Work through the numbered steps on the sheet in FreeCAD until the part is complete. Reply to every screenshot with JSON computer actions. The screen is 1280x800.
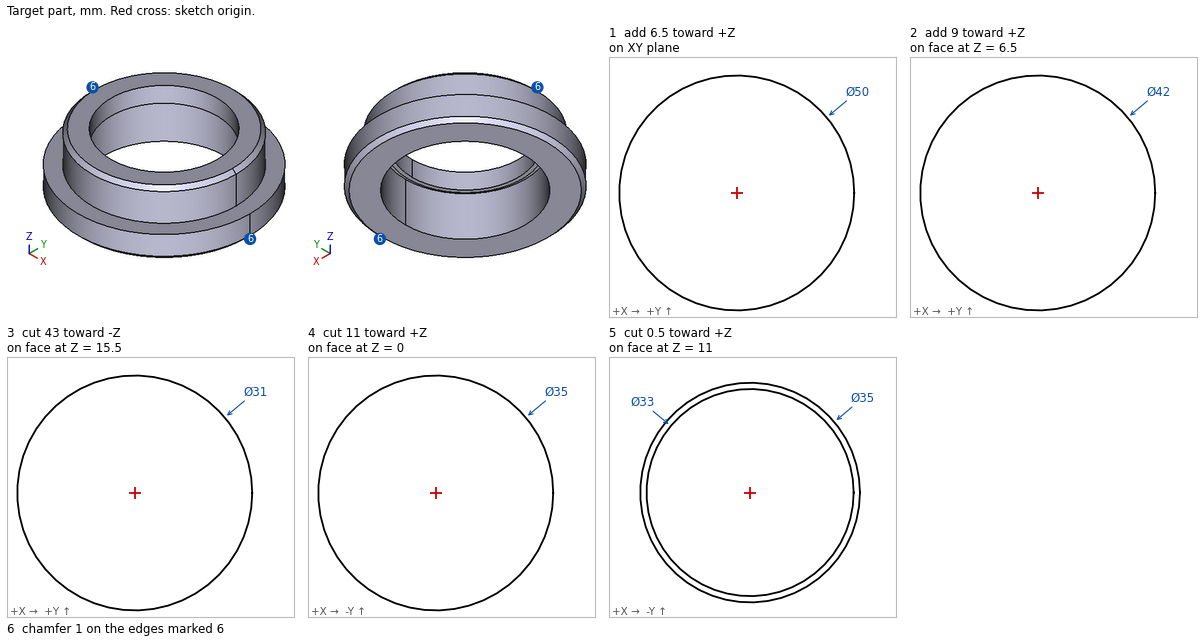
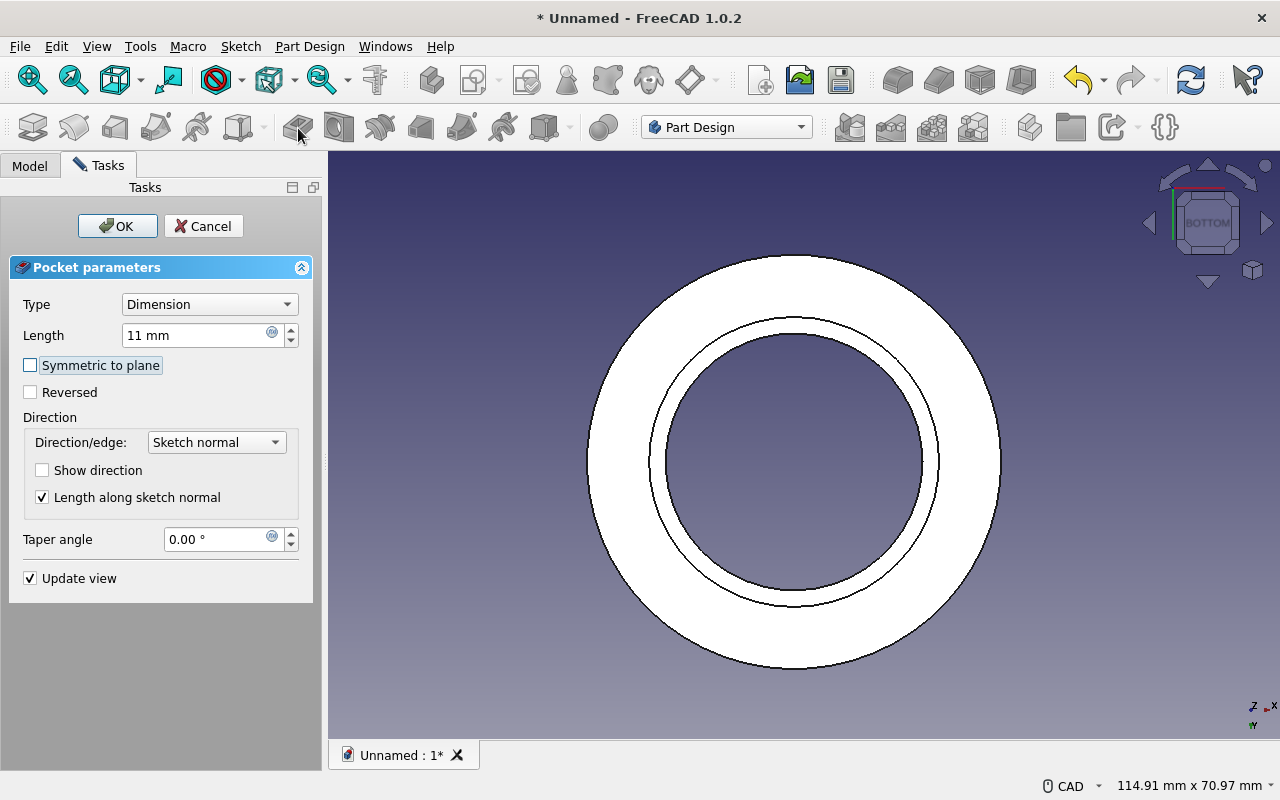
{"action": "left_click", "coordinate": [118, 226]}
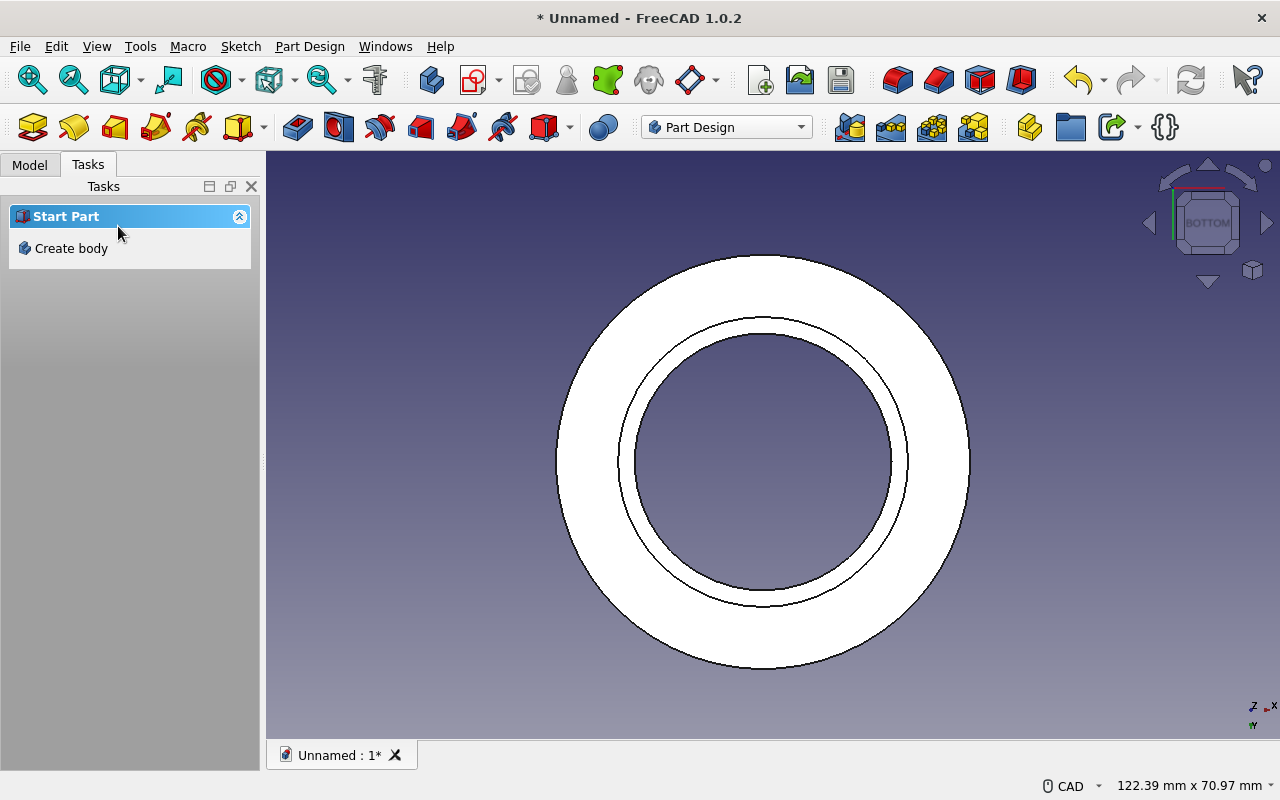
{"action": "scroll", "coordinate": [722, 337], "scroll_direction": "up", "scroll_amount": 8}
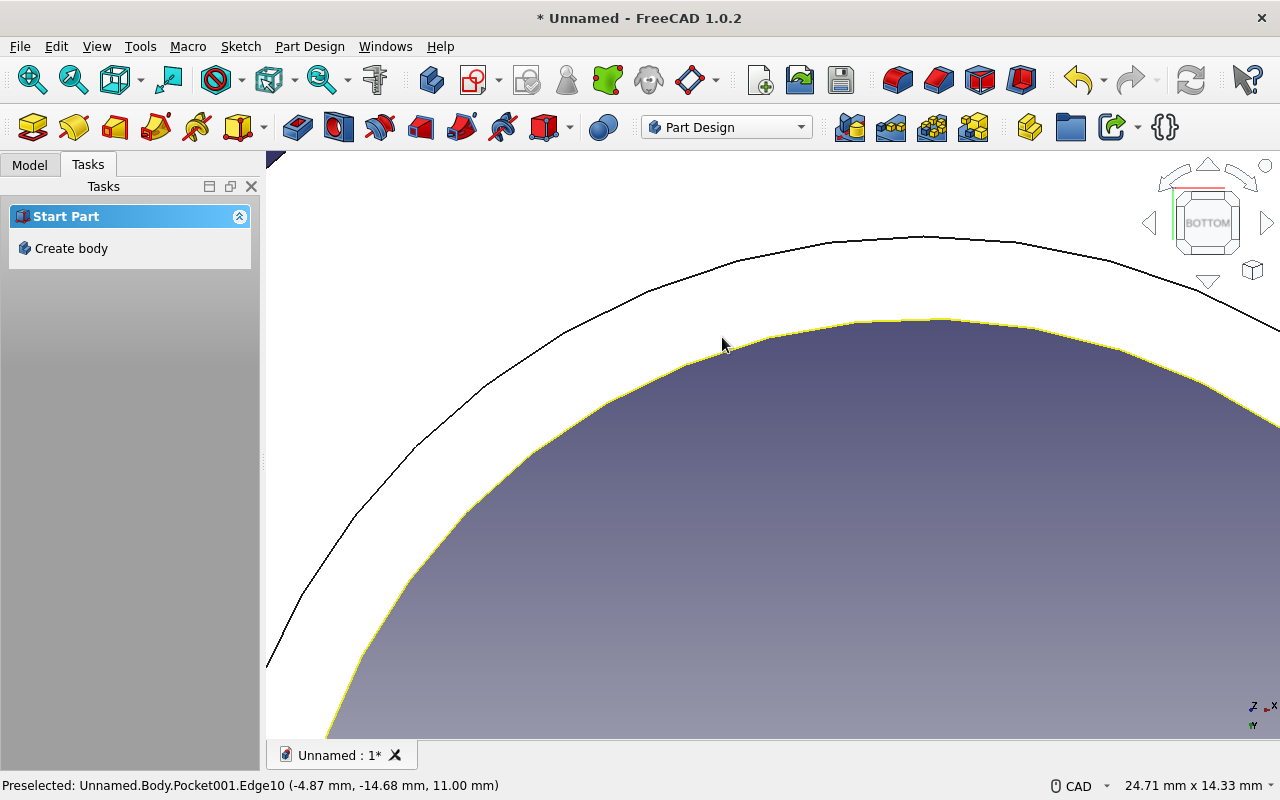
{"action": "left_click", "coordinate": [718, 338]}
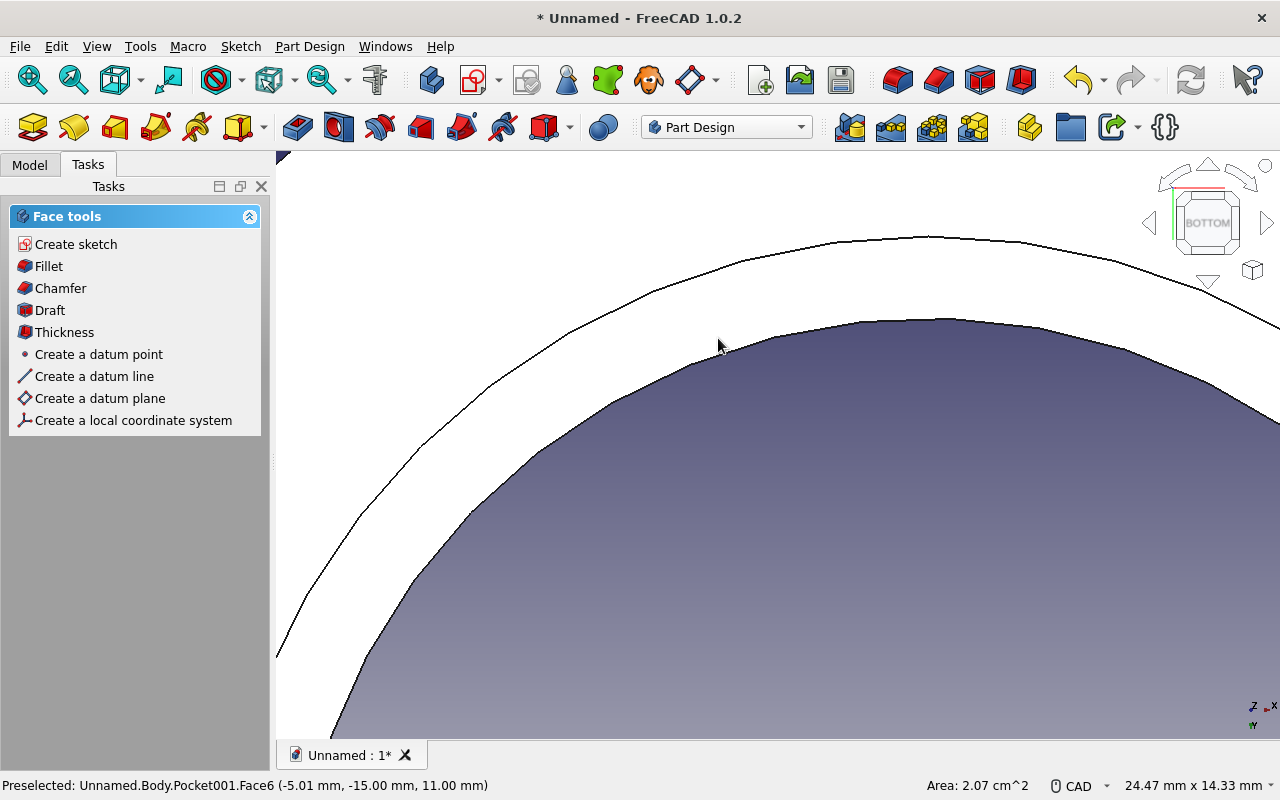
{"action": "left_click", "coordinate": [472, 80]}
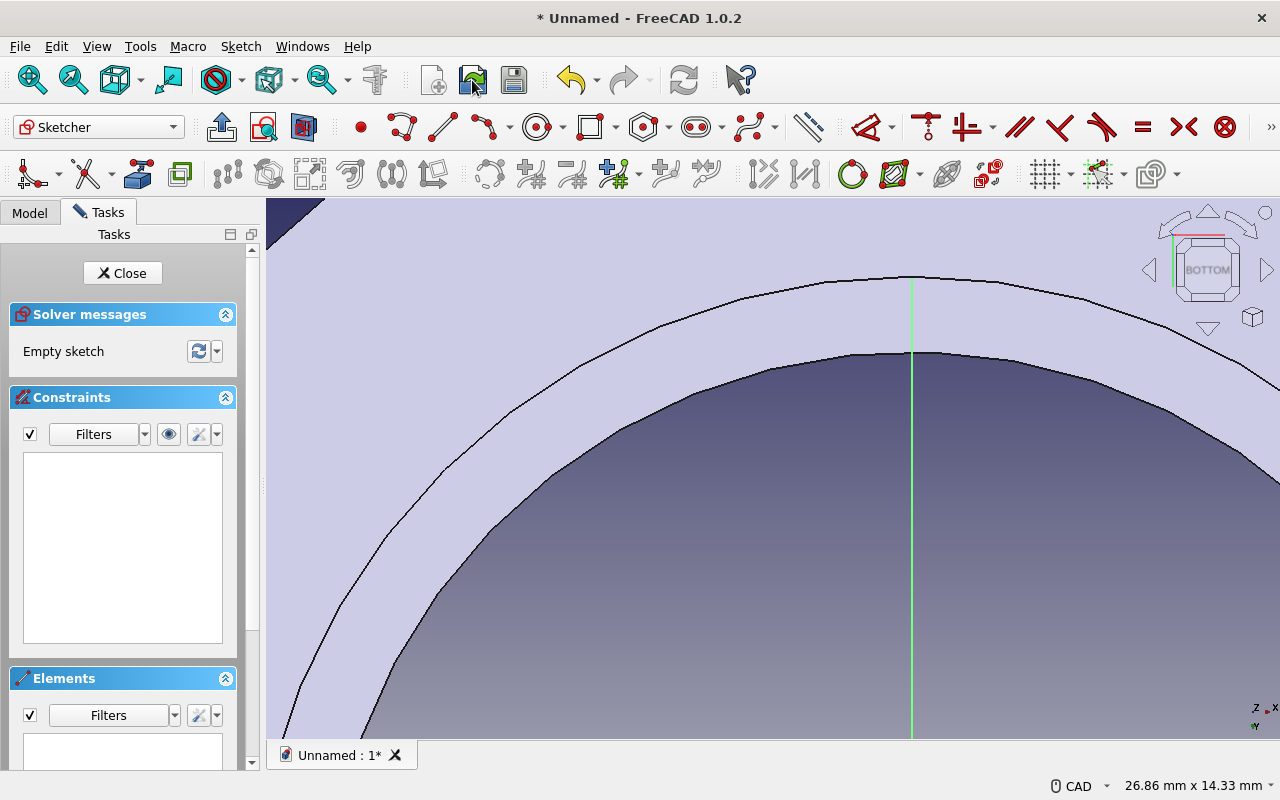
{"action": "left_click", "coordinate": [304, 128]}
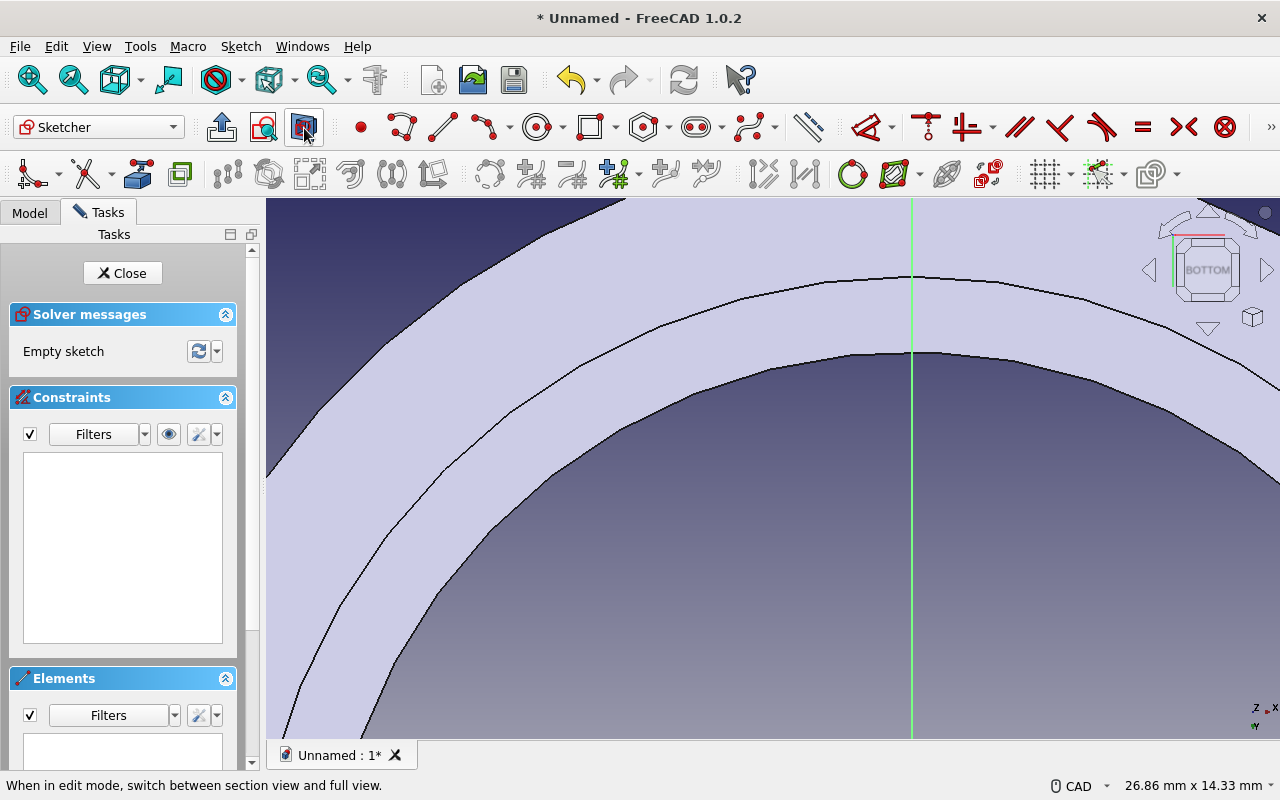
{"action": "scroll", "coordinate": [637, 315], "scroll_direction": "down", "scroll_amount": 7}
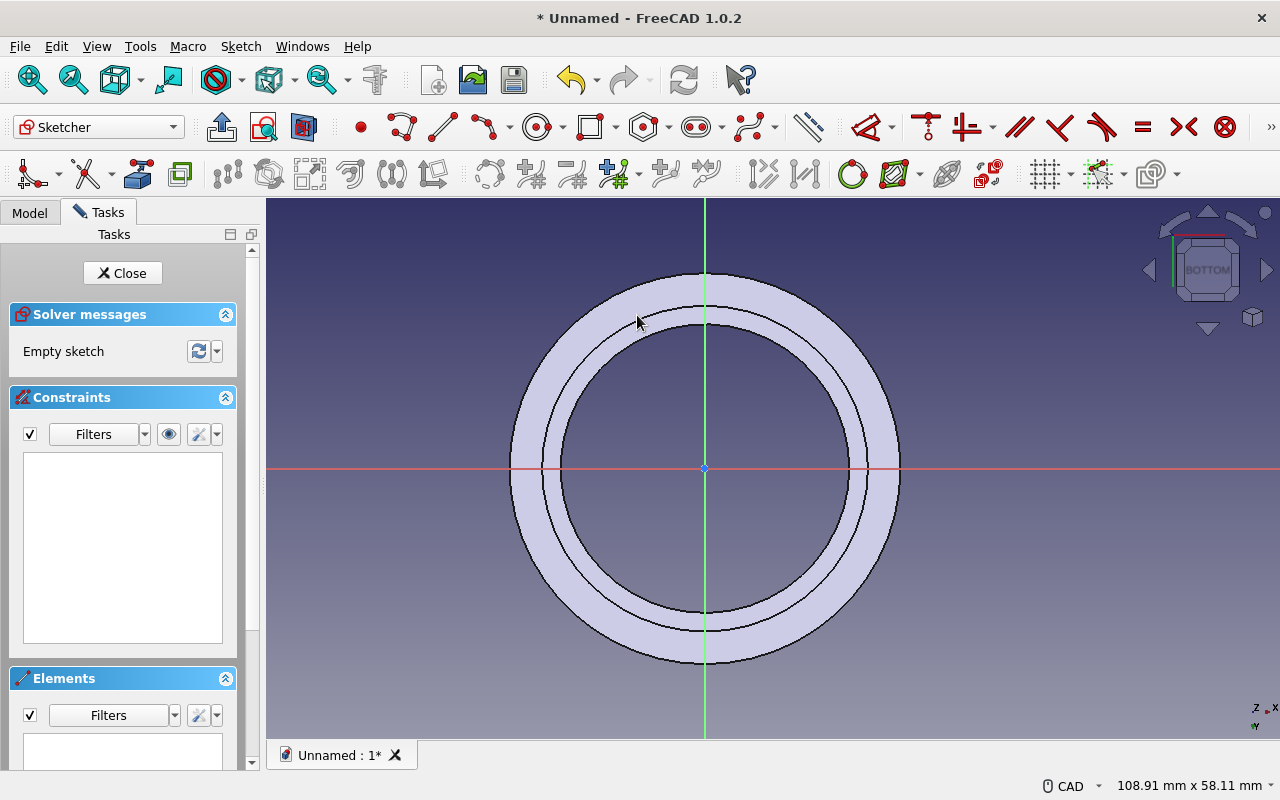
{"action": "left_click", "coordinate": [536, 128]}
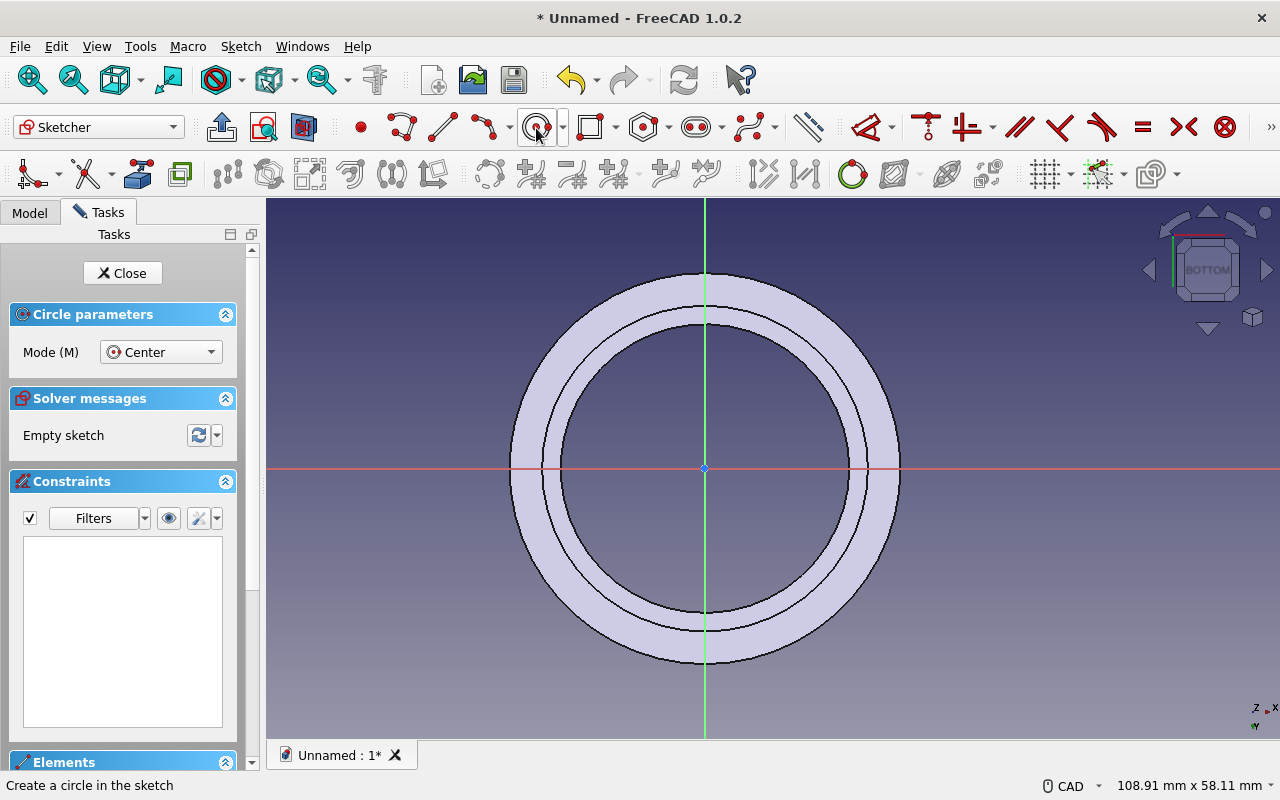
{"action": "left_click", "coordinate": [705, 469]}
{"action": "mouse_move", "coordinate": [820, 353]}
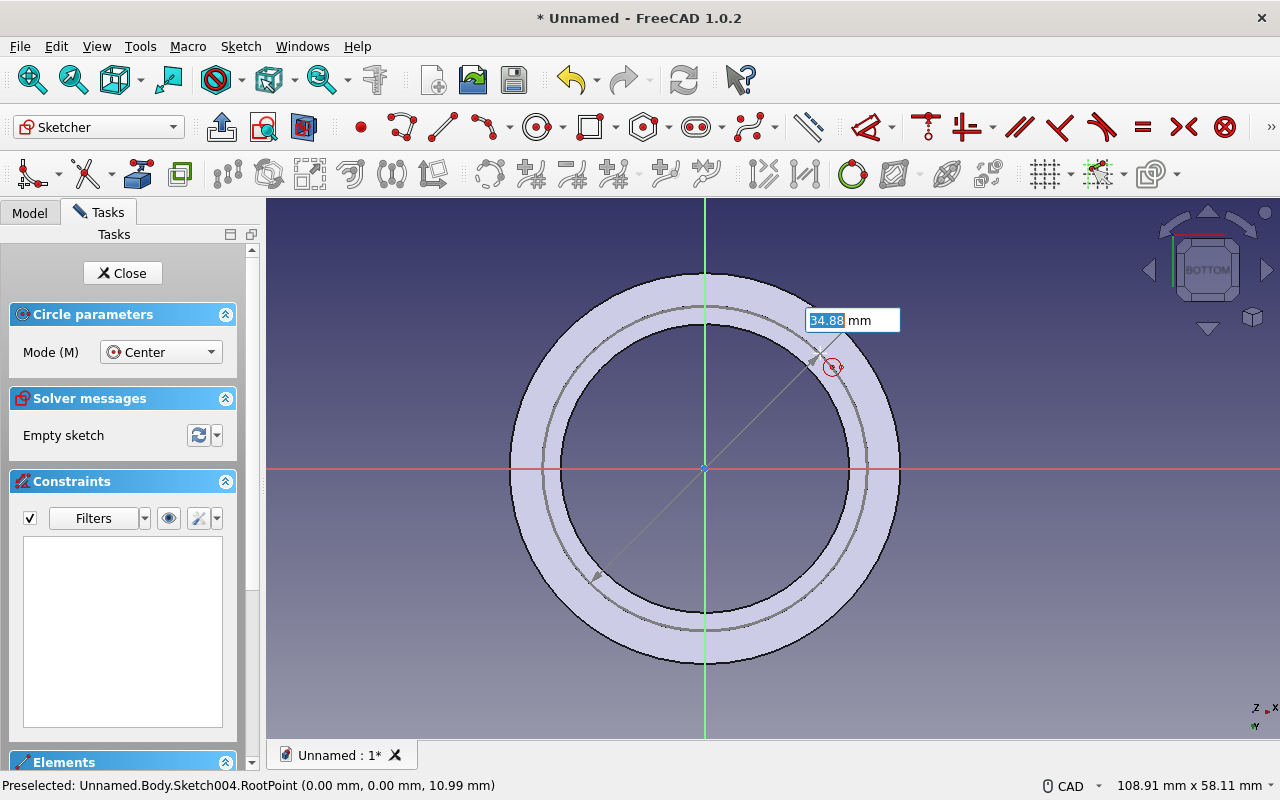
{"action": "type", "text": "35"}
{"action": "key", "text": "Return"}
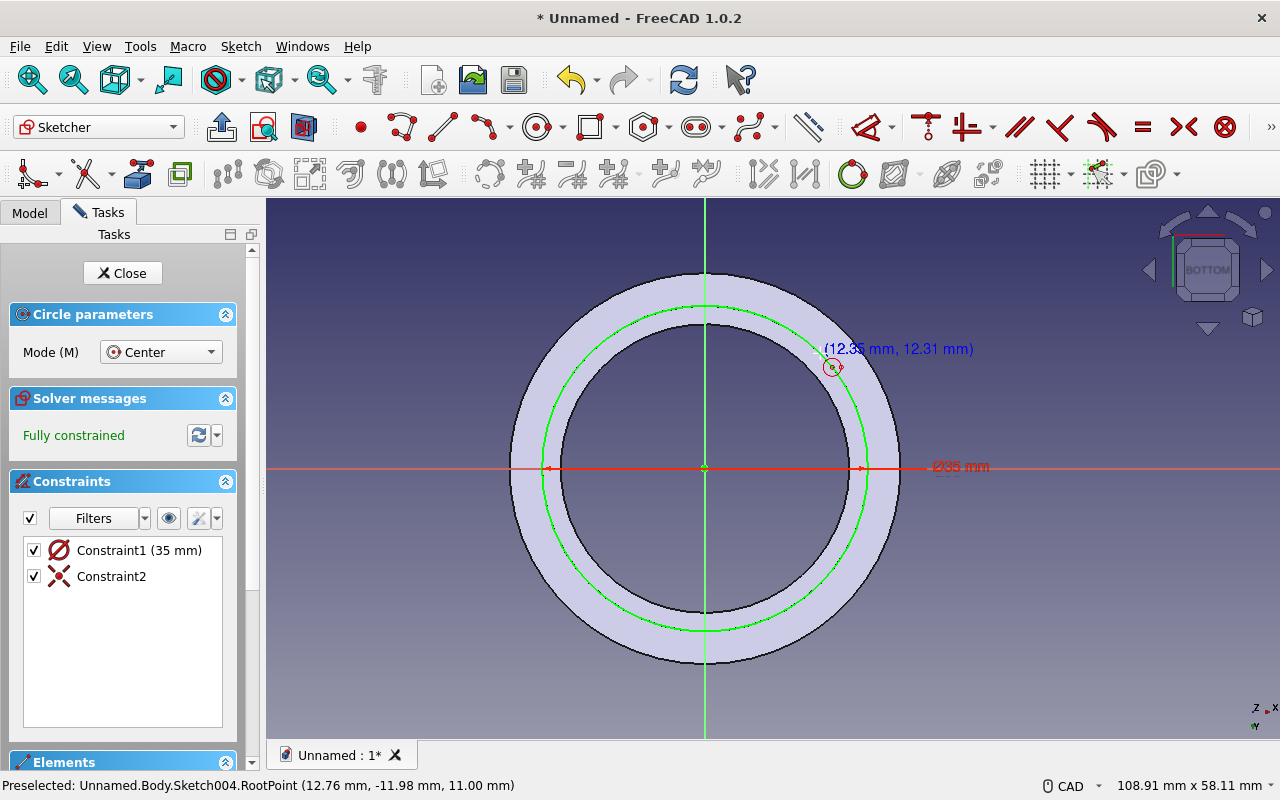
{"action": "left_click", "coordinate": [705, 469]}